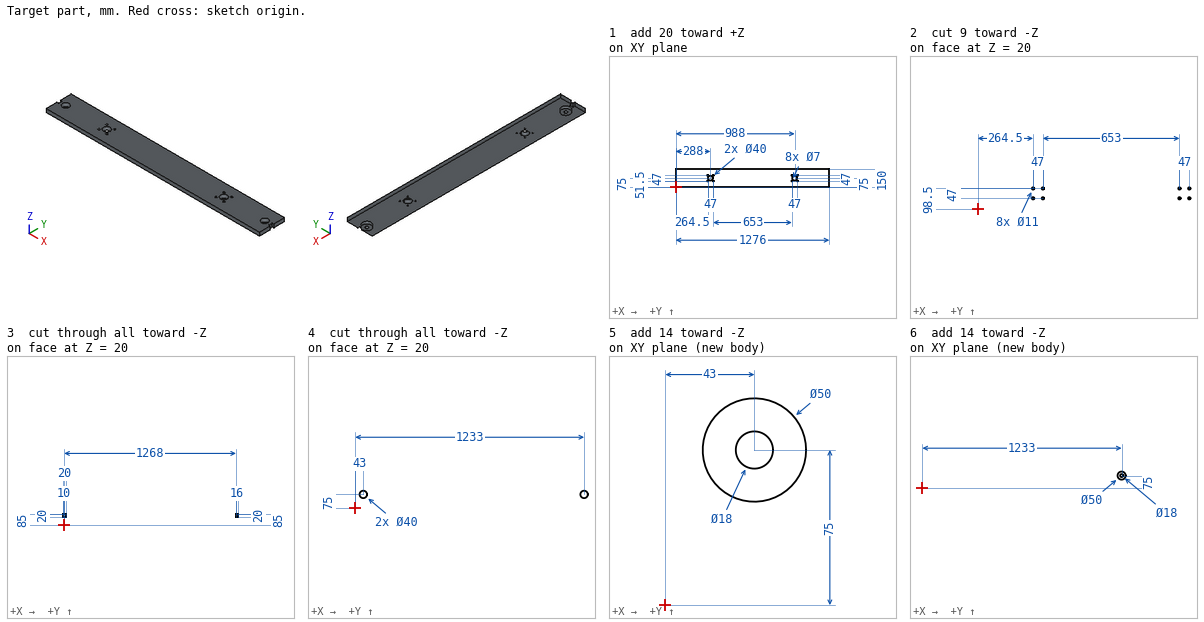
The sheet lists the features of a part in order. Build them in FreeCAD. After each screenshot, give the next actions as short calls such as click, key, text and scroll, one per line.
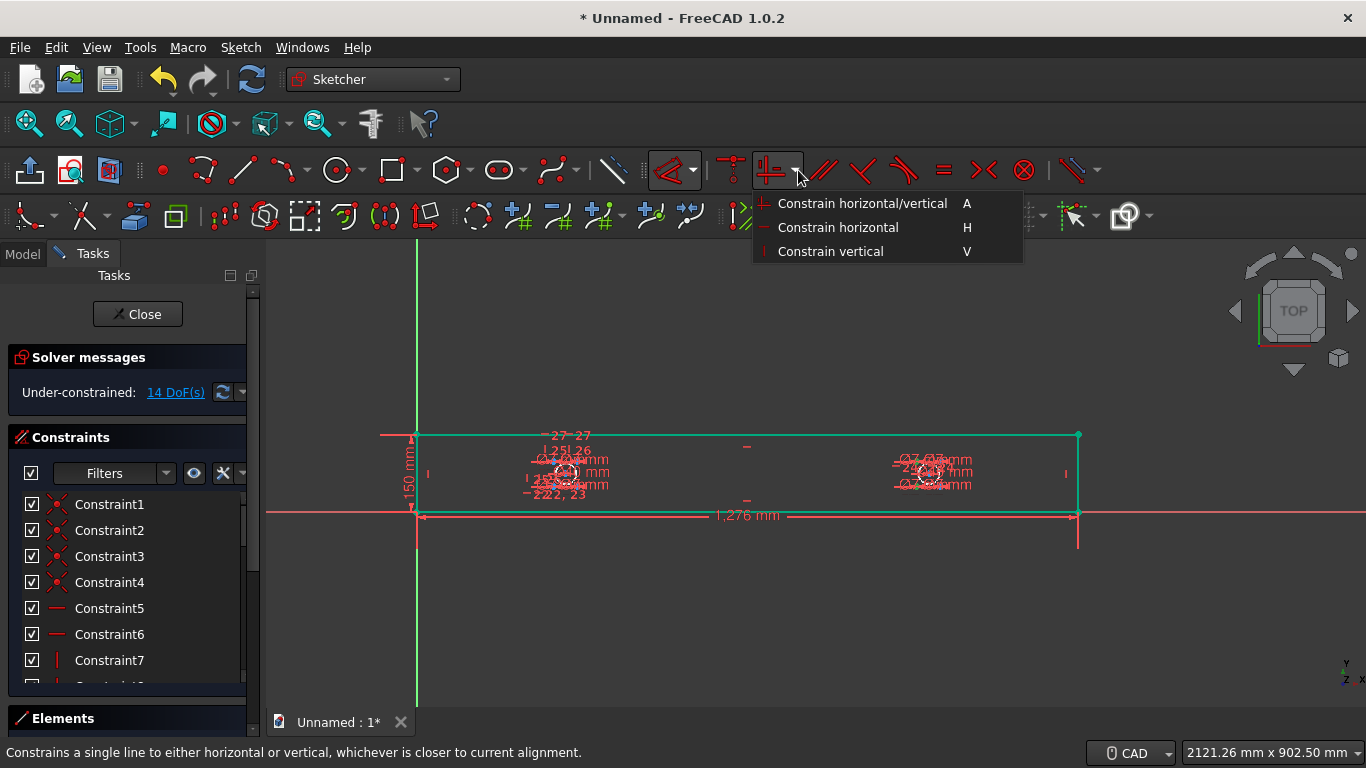
click(888, 251)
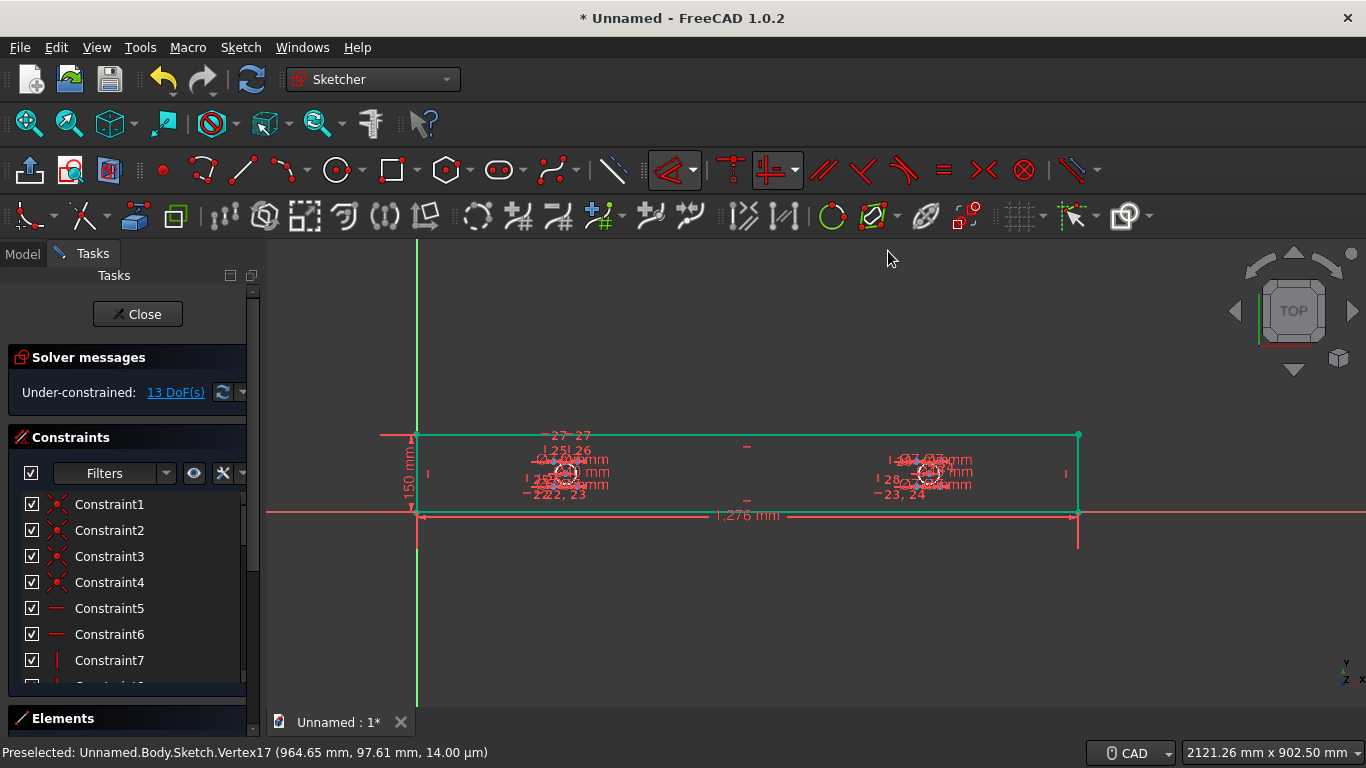
click(941, 487)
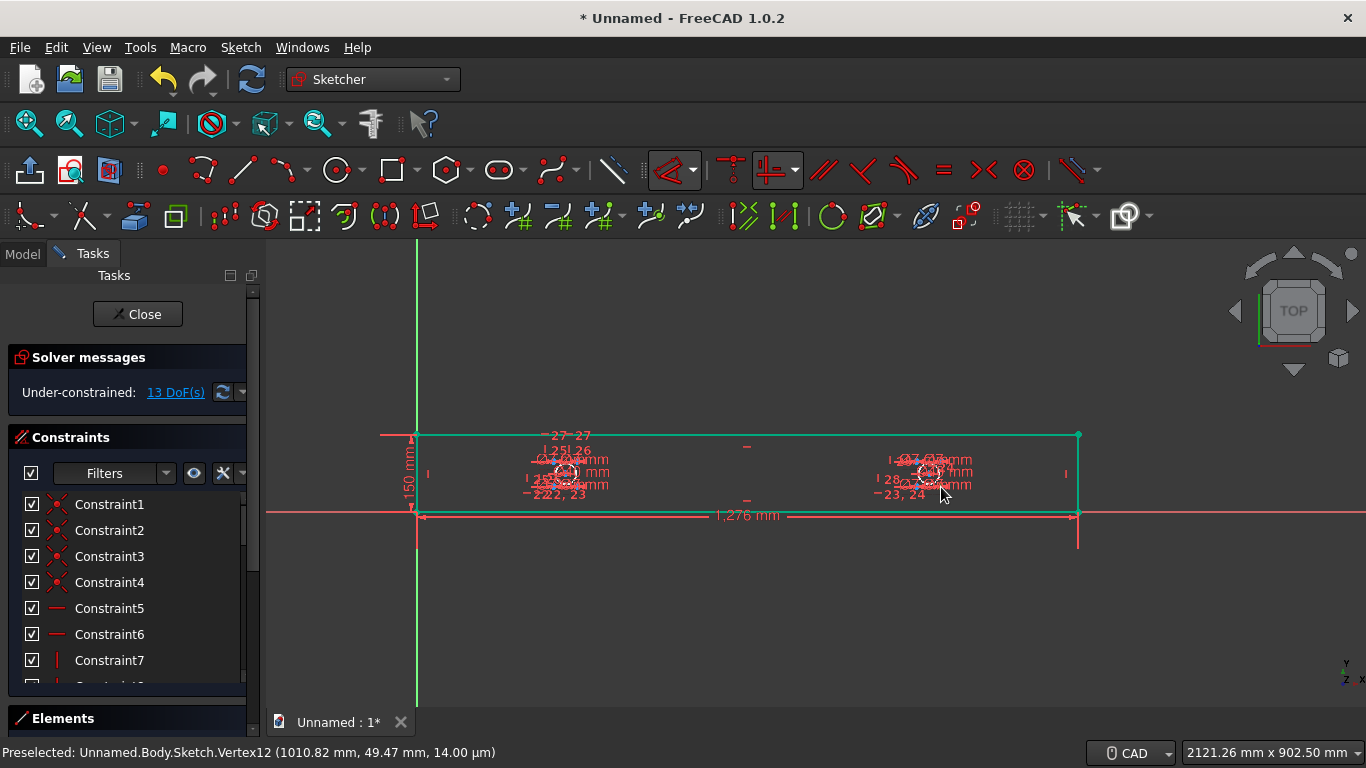
scroll(941, 462, up, 4)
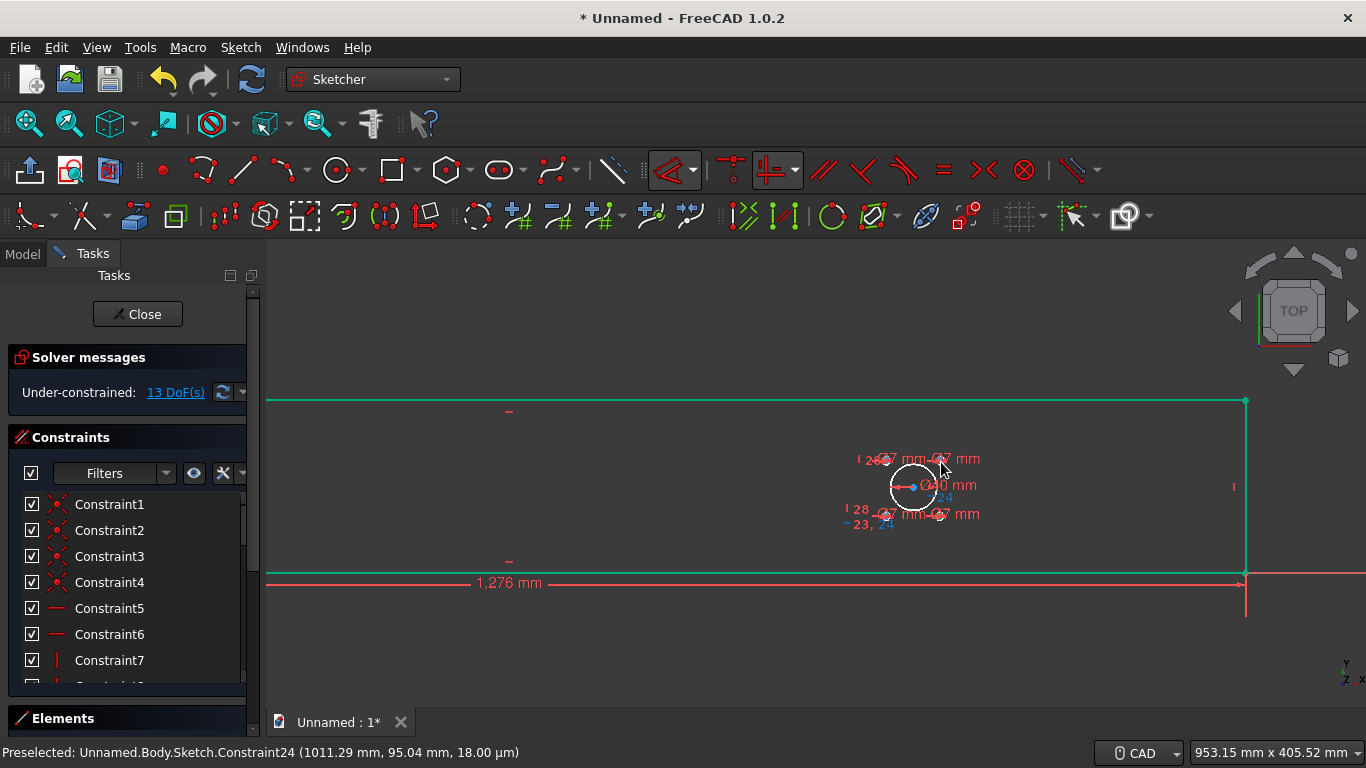
click(940, 461)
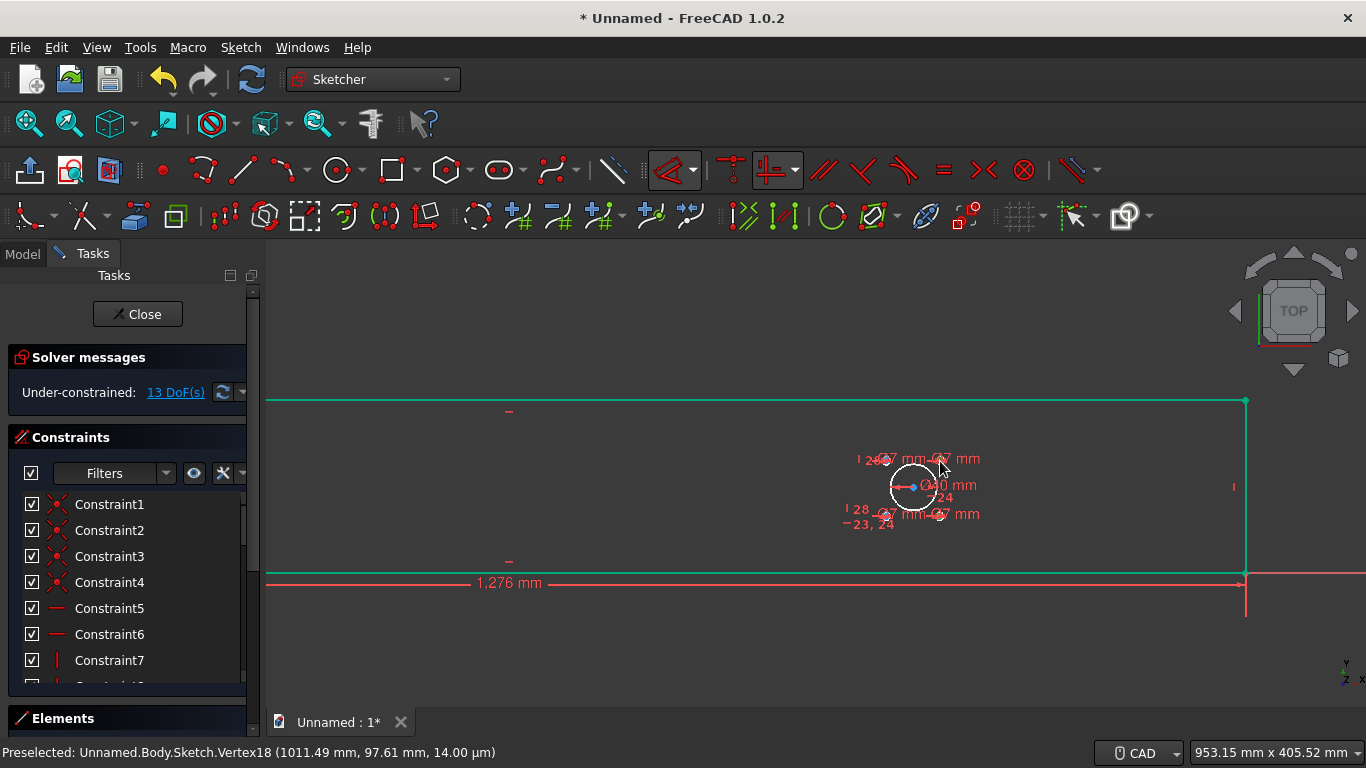
key(v)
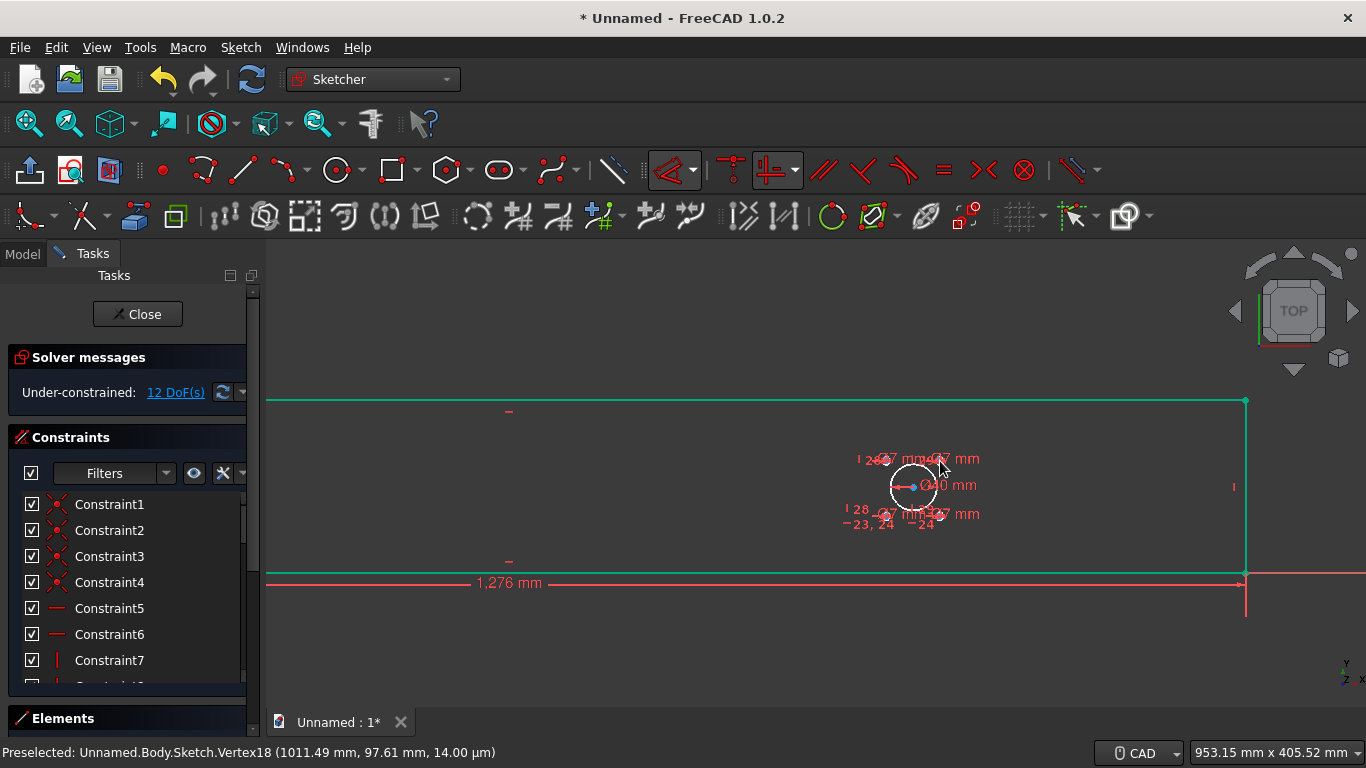
click(886, 461)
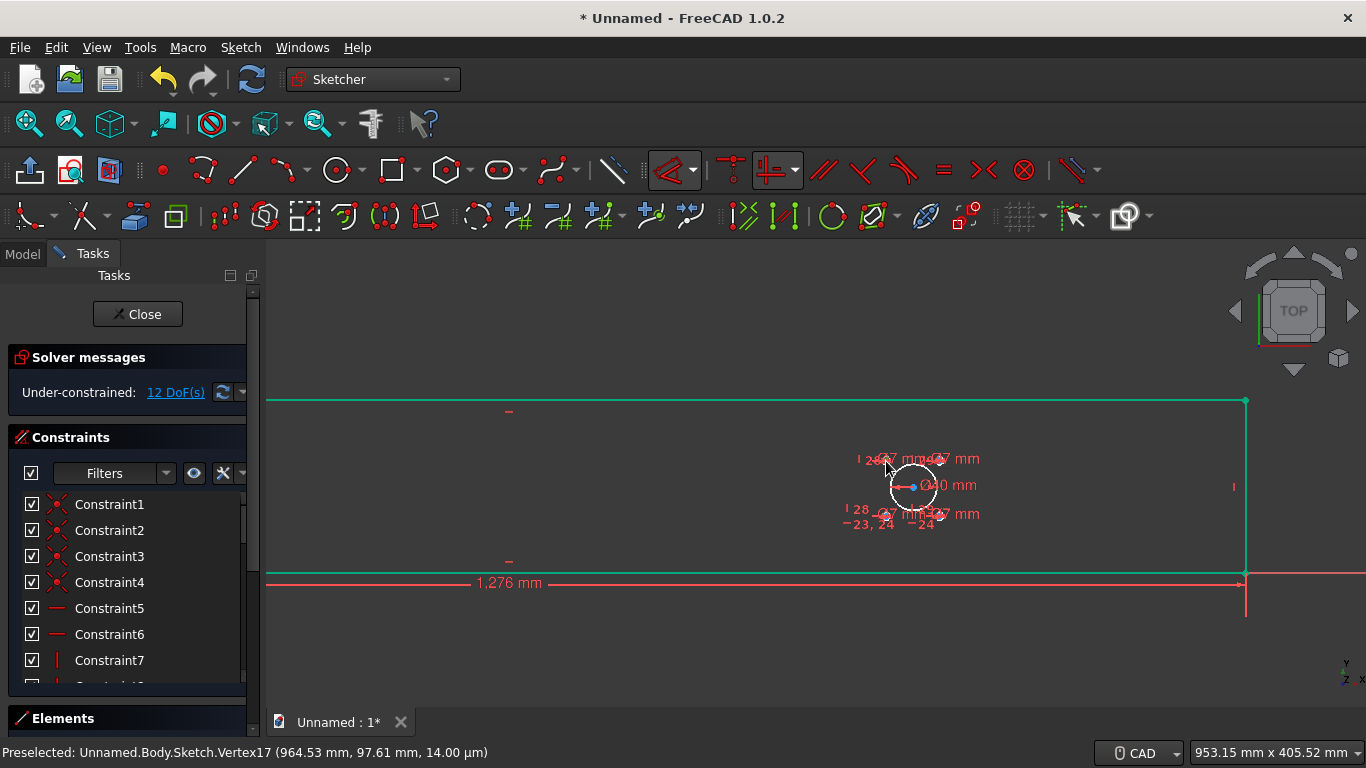
click(940, 461)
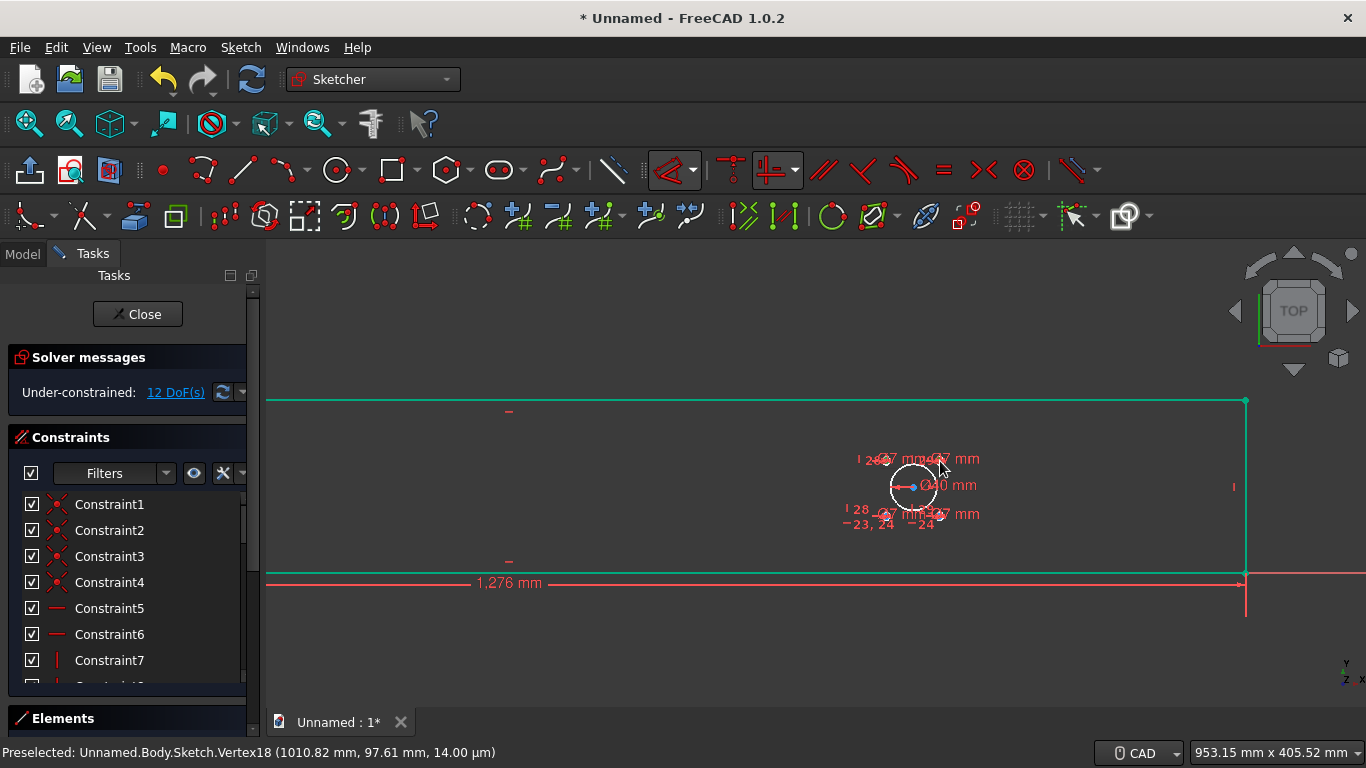
key(h)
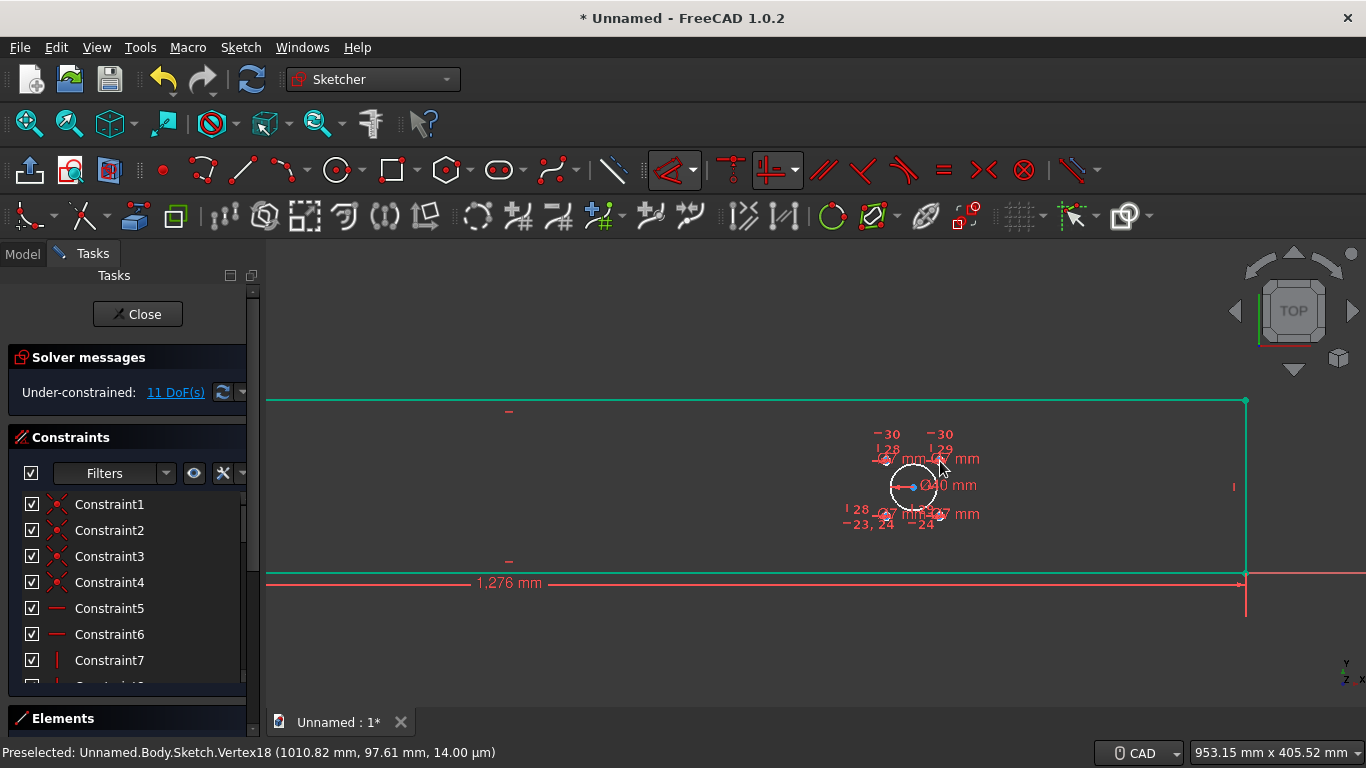
click(668, 170)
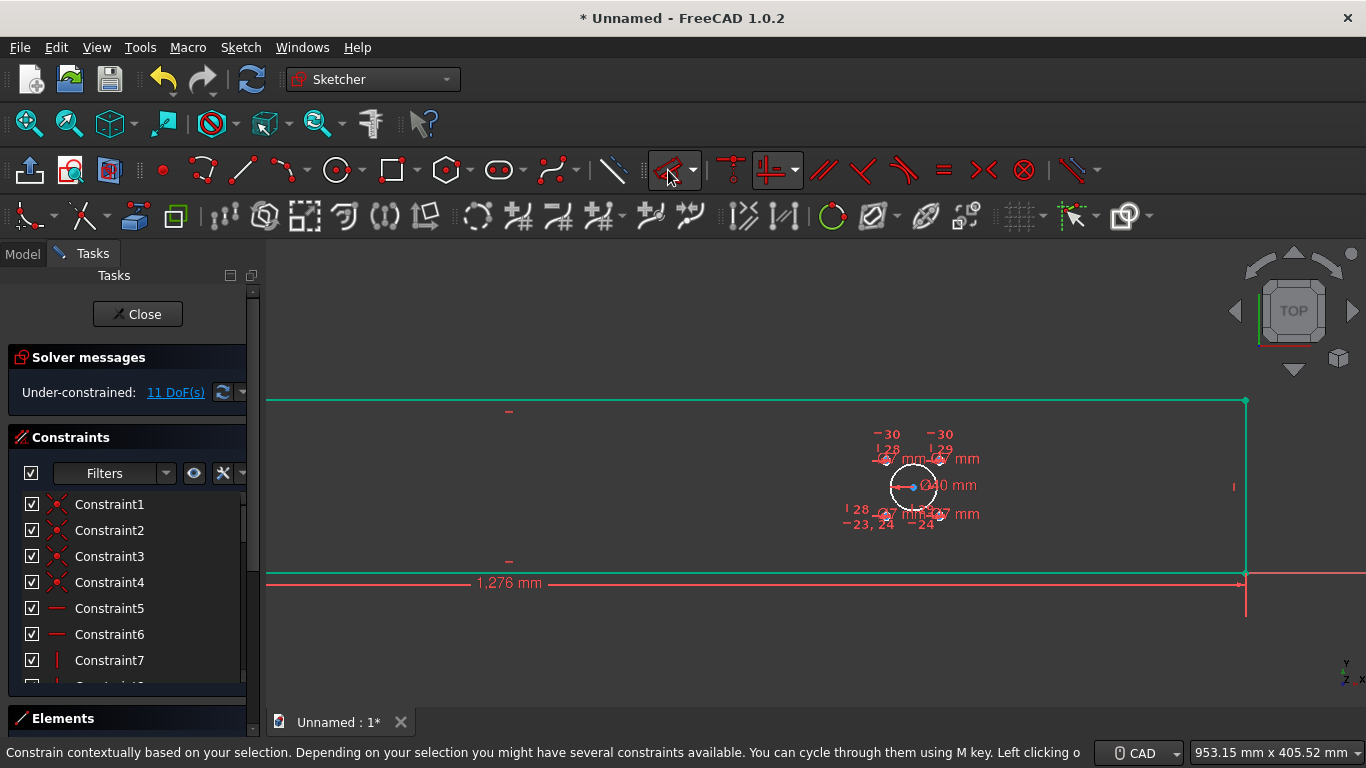
scroll(942, 462, down, 4)